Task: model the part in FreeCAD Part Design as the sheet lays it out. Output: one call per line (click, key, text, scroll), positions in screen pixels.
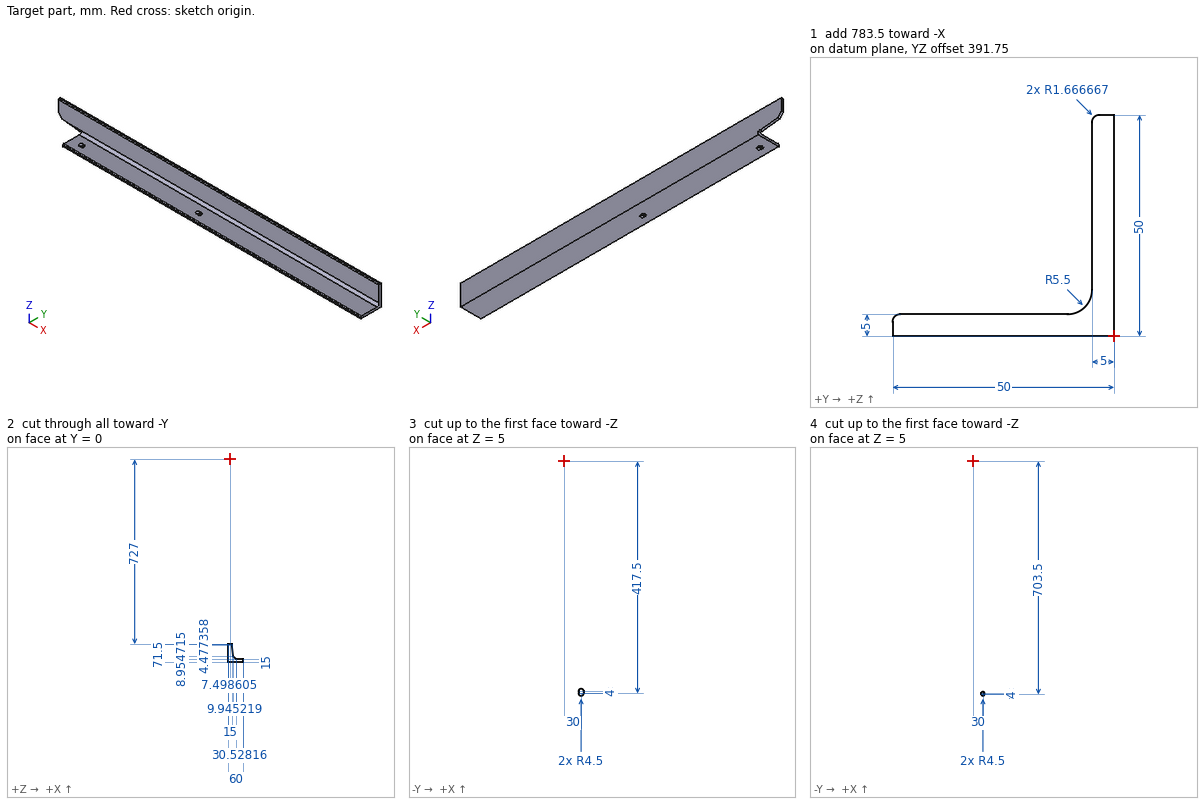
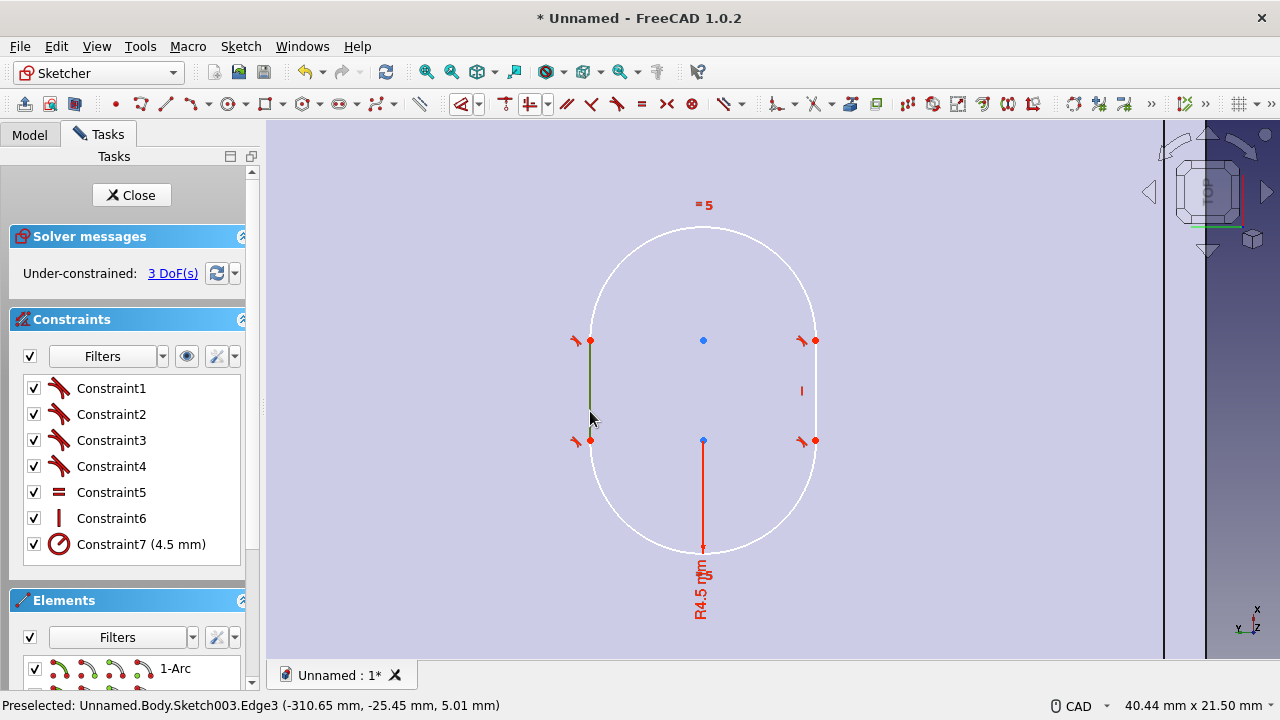
click(478, 104)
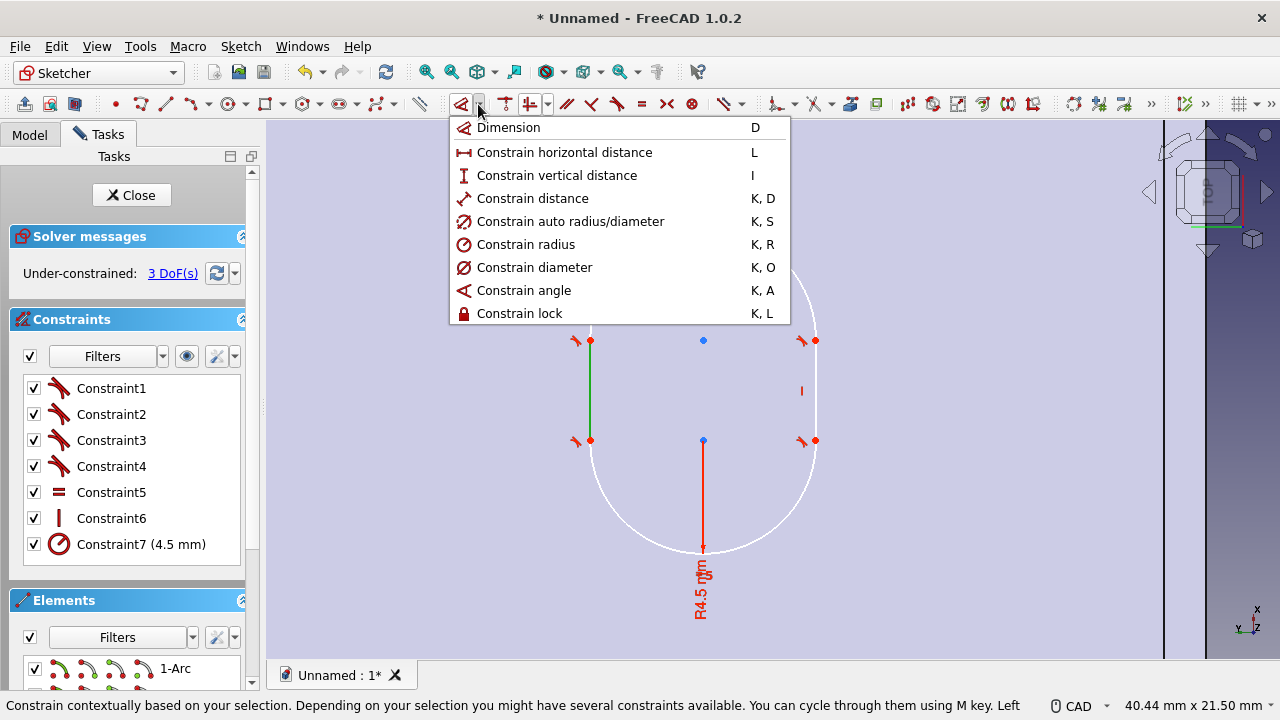
click(620, 176)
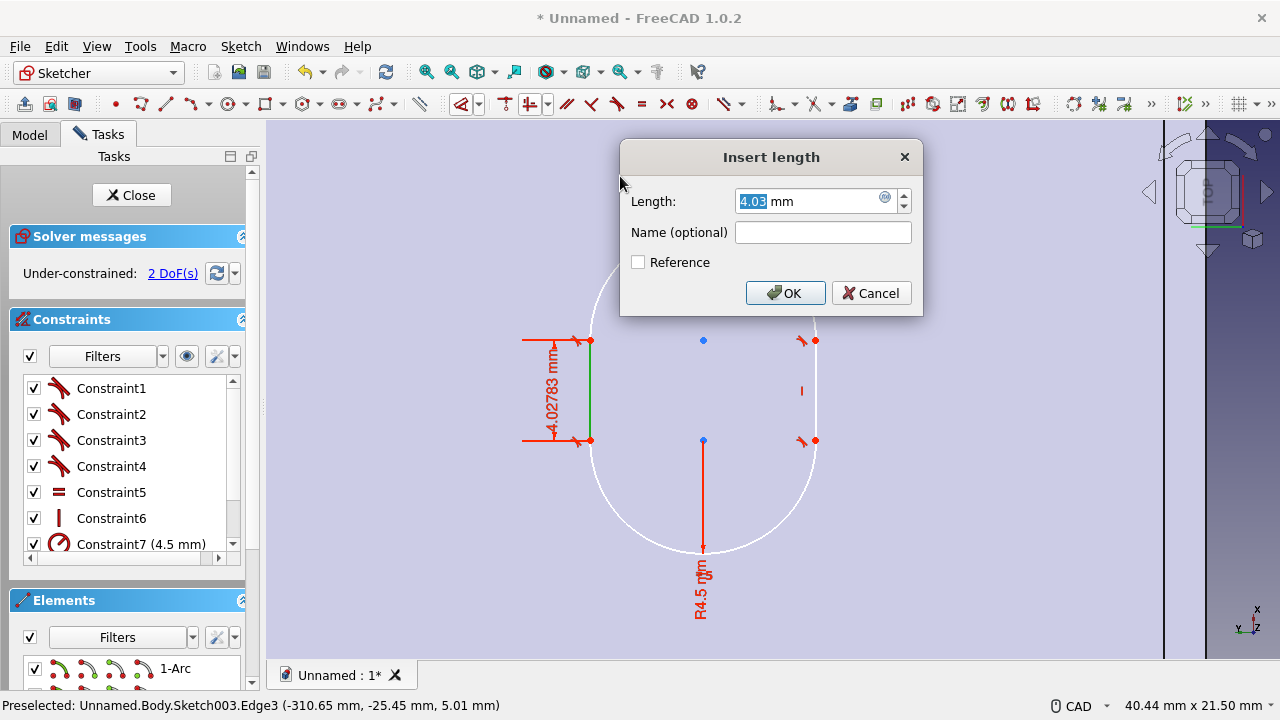
text(4)
key(Return)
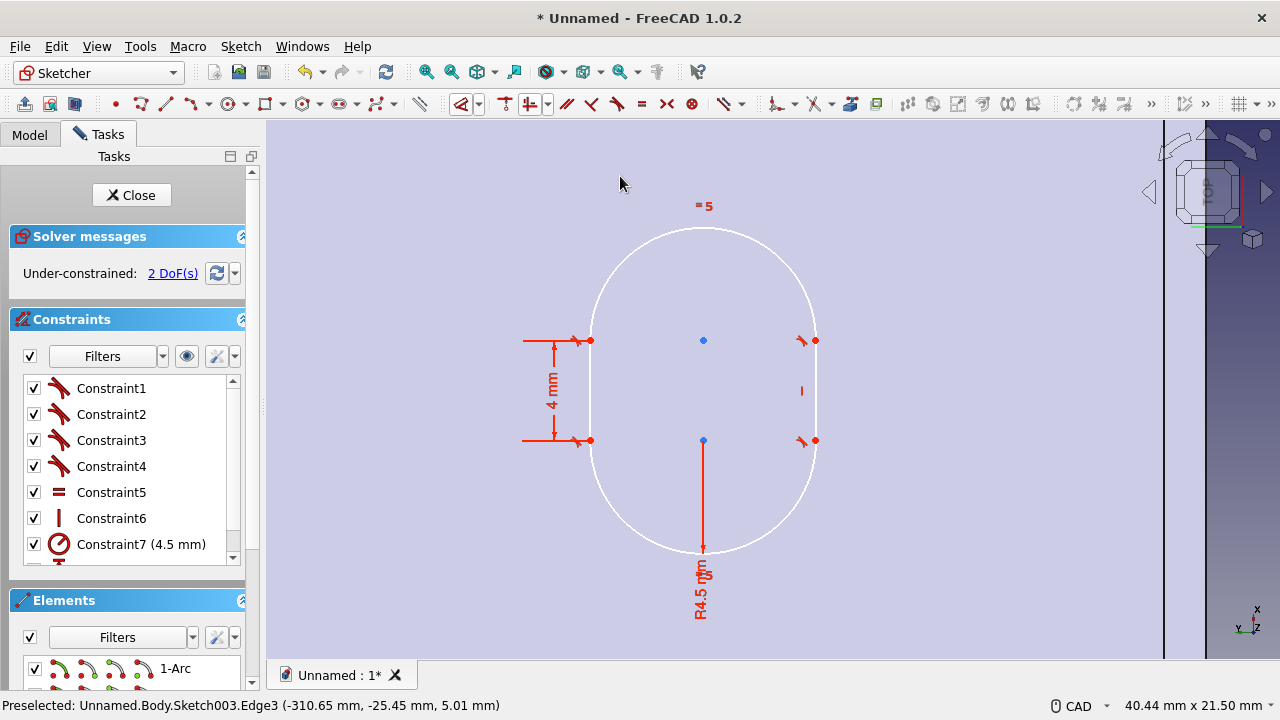
click(703, 441)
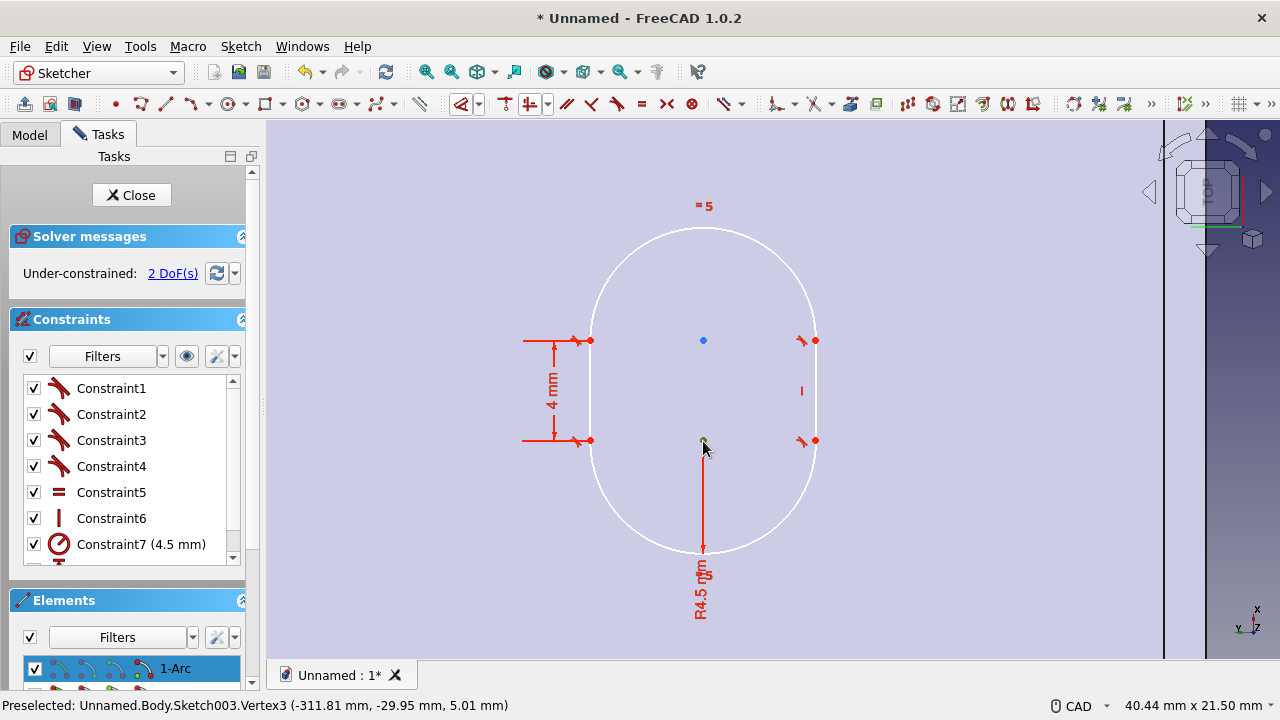
key(l)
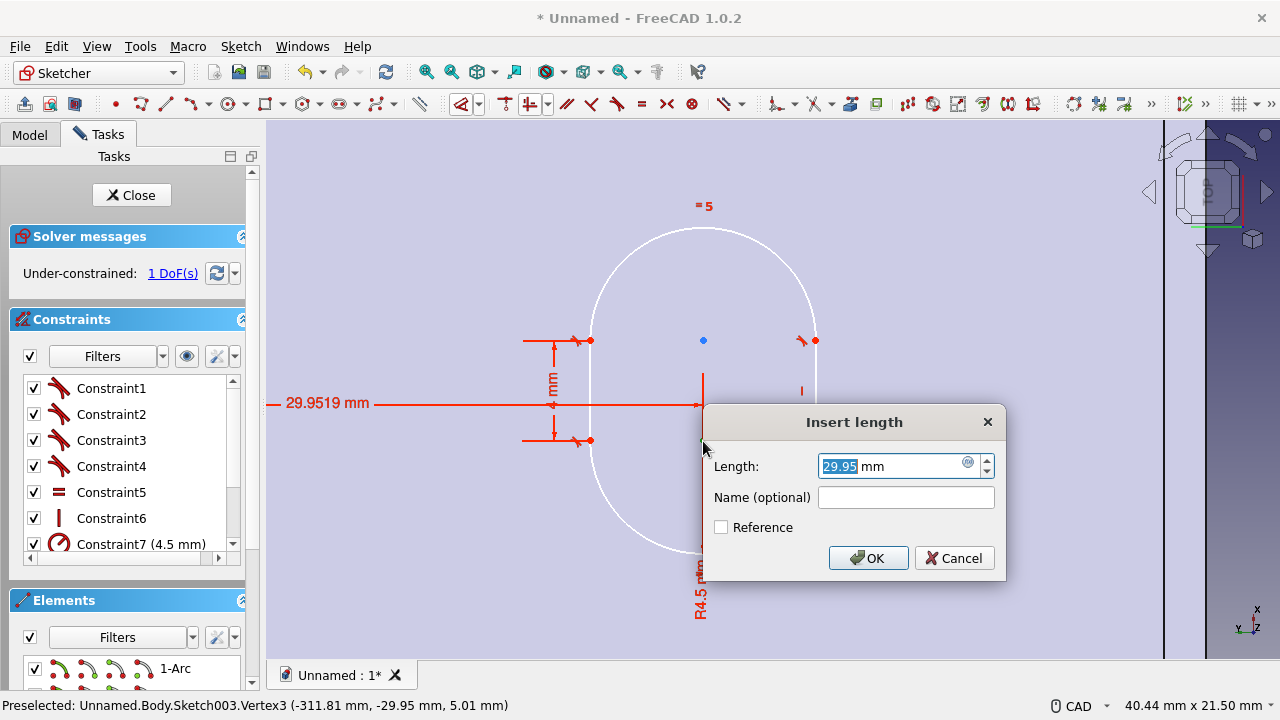
text(30)
key(Return)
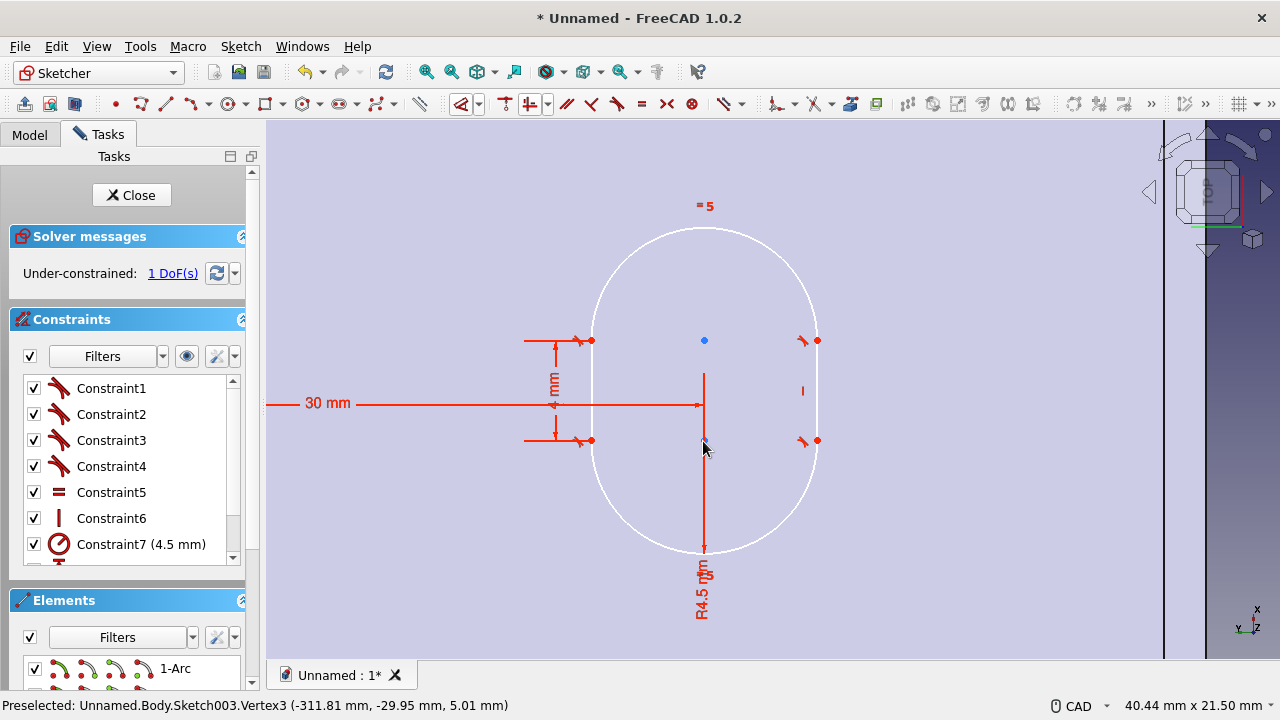
click(592, 441)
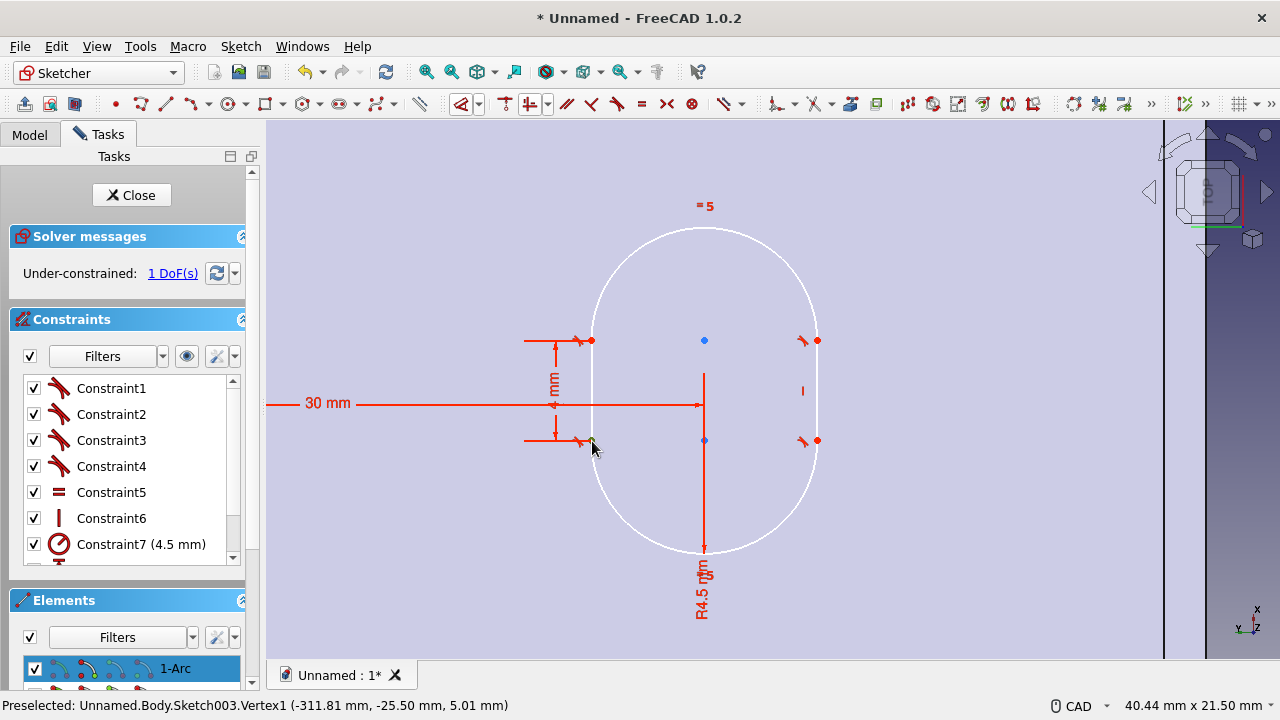
key(i)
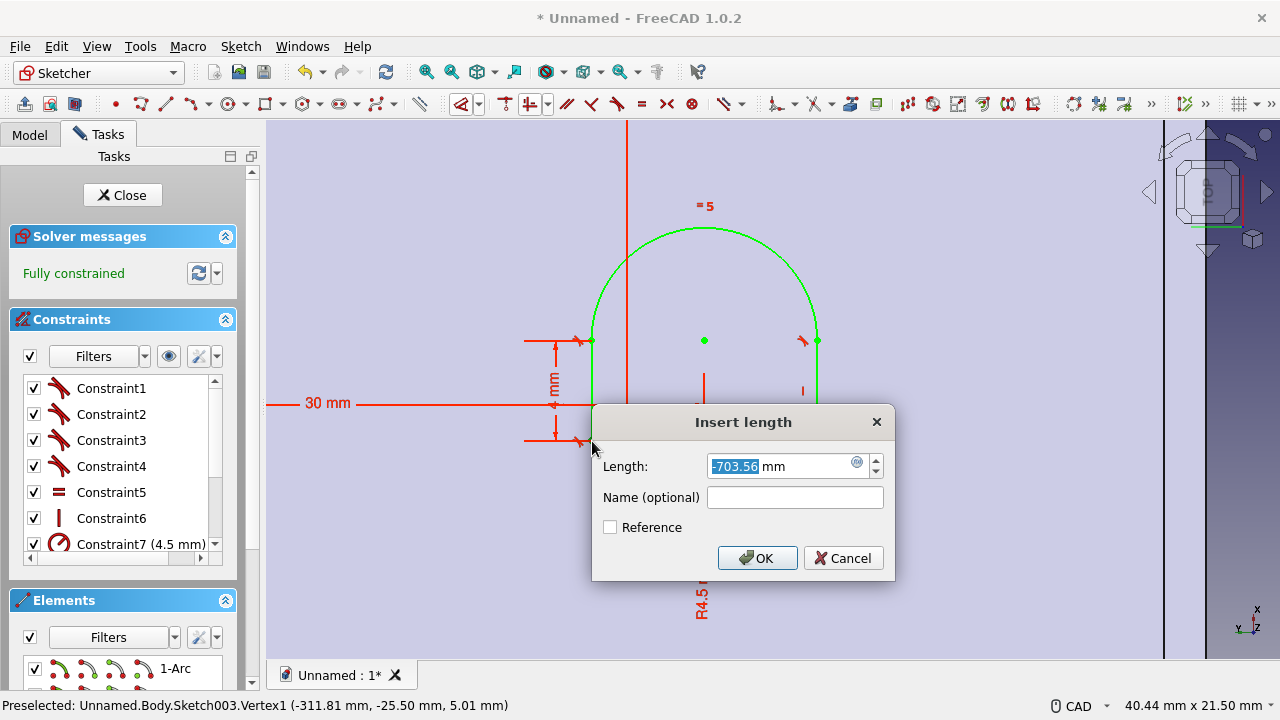
text(-703.5)
key(Return)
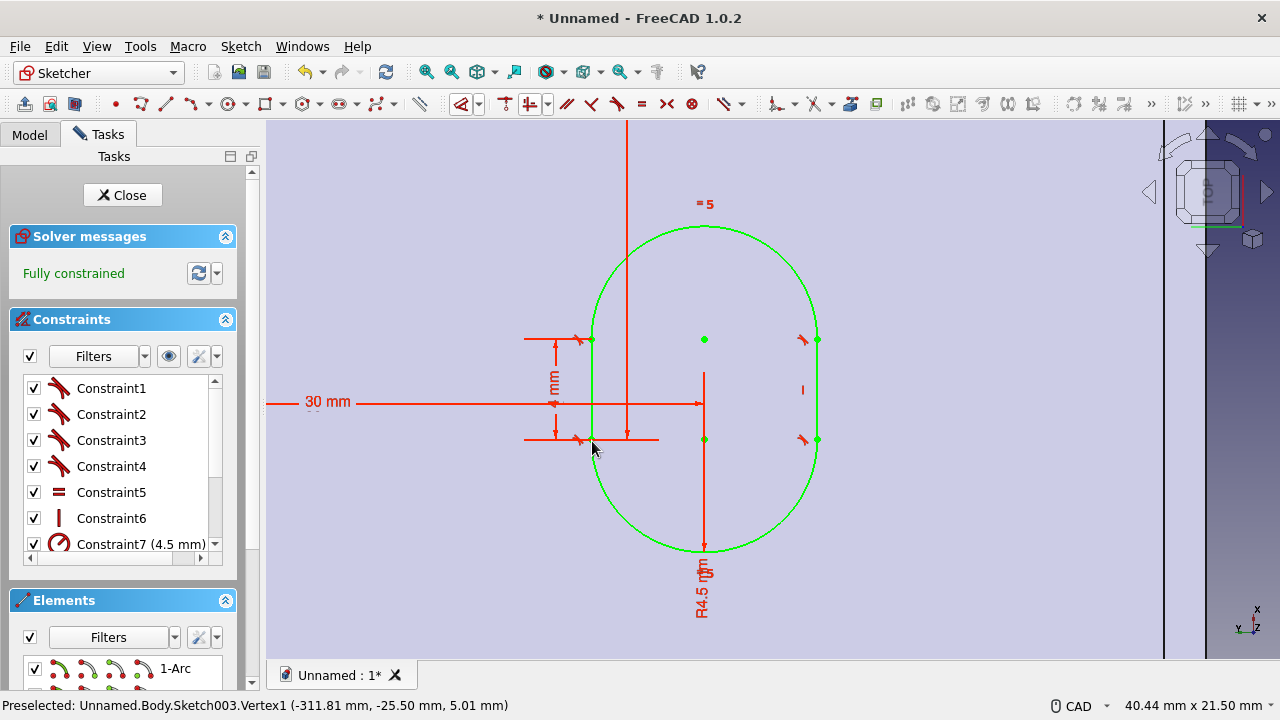
click(123, 195)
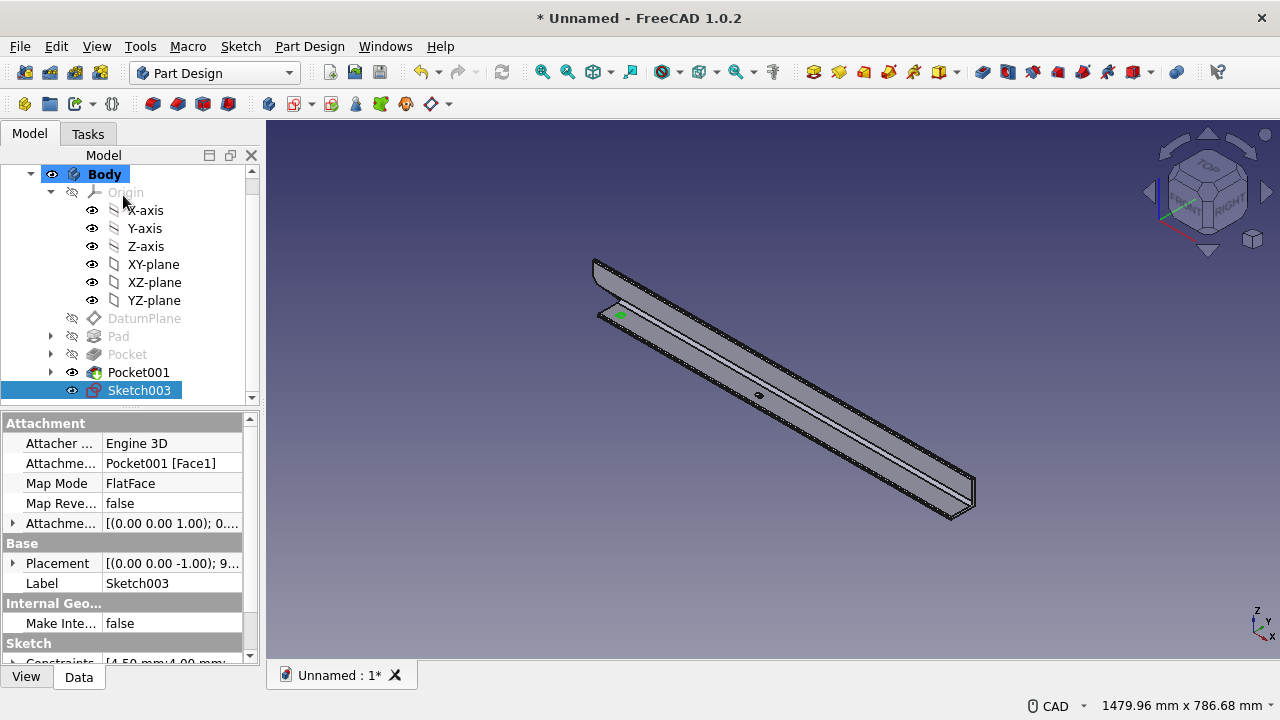
click(983, 72)